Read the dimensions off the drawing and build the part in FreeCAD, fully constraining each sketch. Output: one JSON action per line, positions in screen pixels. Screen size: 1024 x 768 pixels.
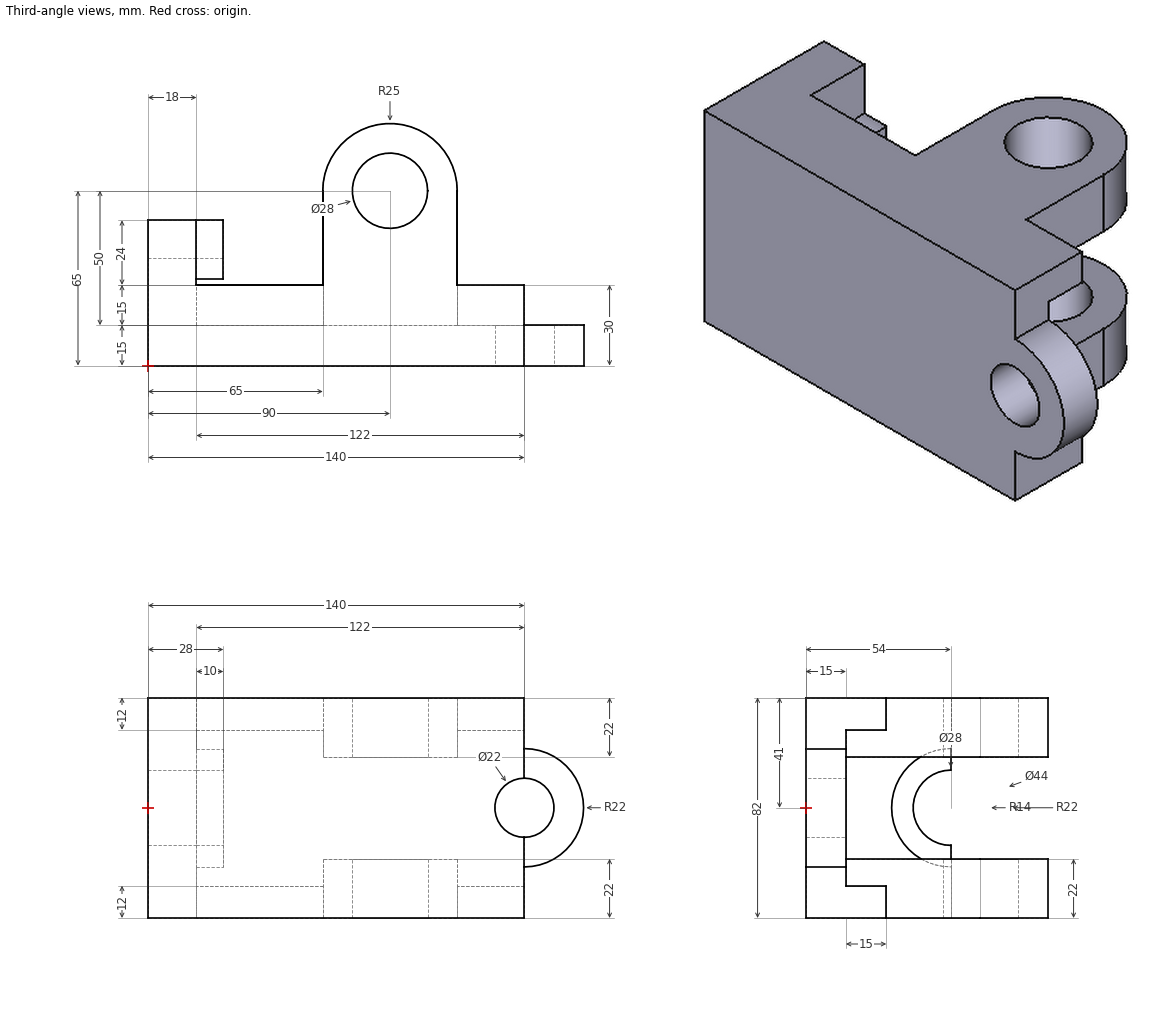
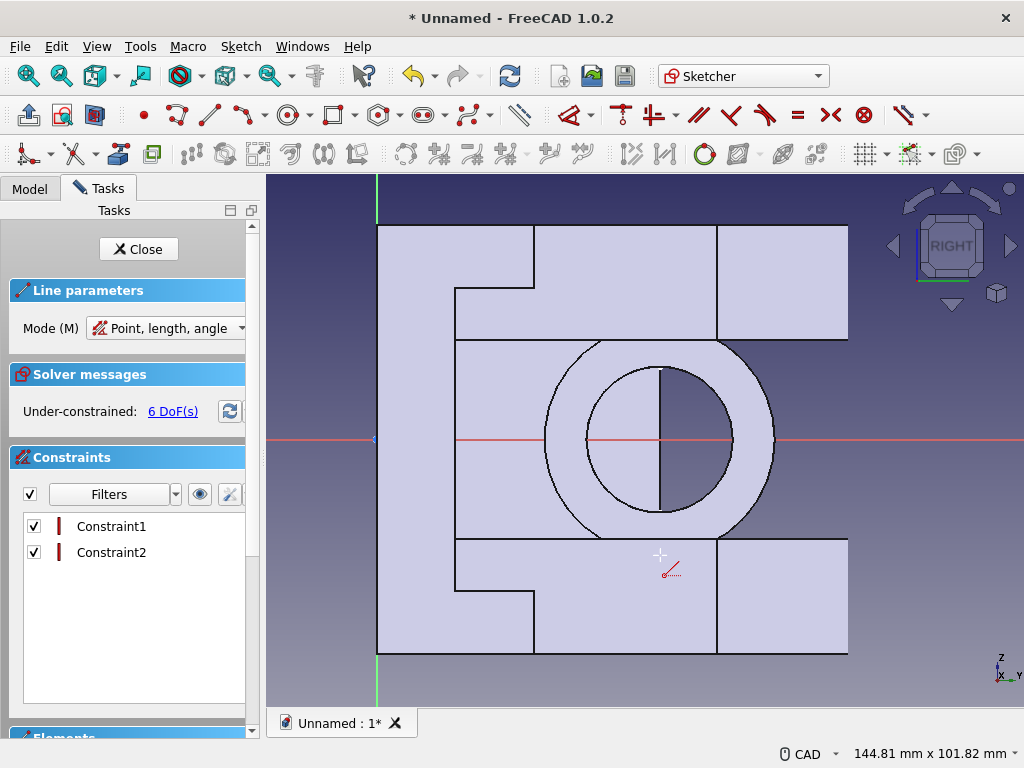
{"action": "key", "text": "g 3 a"}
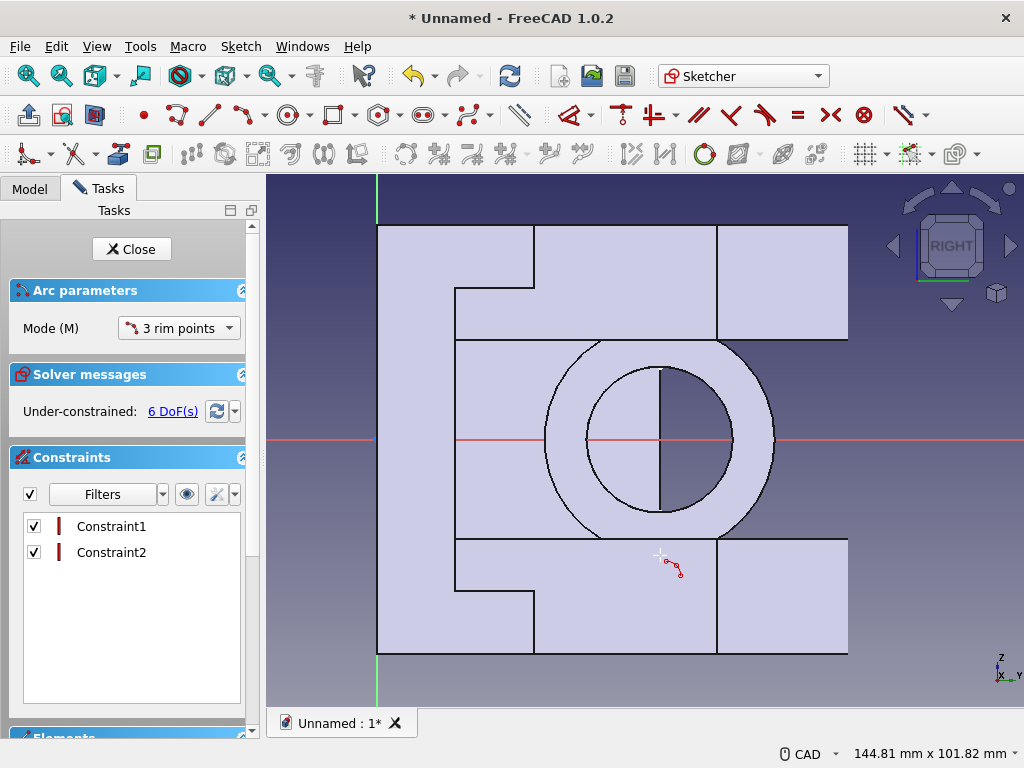
{"action": "left_click", "coordinate": [660, 367]}
{"action": "left_click", "coordinate": [660, 514]}
{"action": "left_click", "coordinate": [729, 462]}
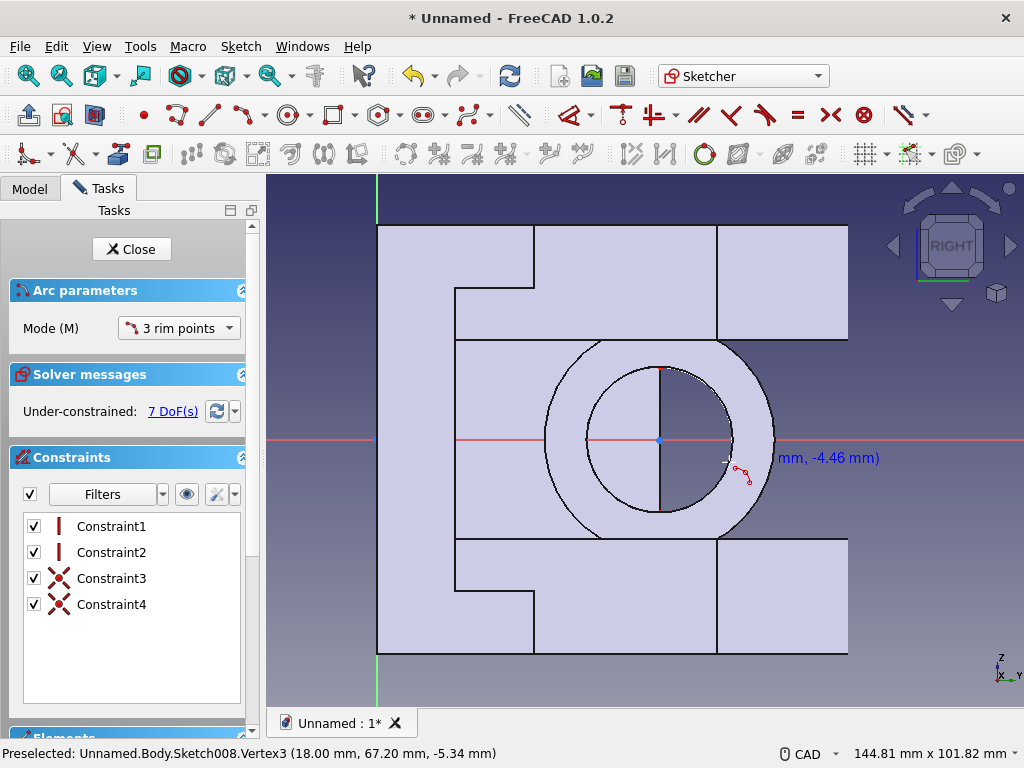
{"action": "left_click", "coordinate": [660, 556]}
{"action": "left_click", "coordinate": [660, 326]}
{"action": "left_click", "coordinate": [769, 475]}
{"action": "key", "text": "Escape"}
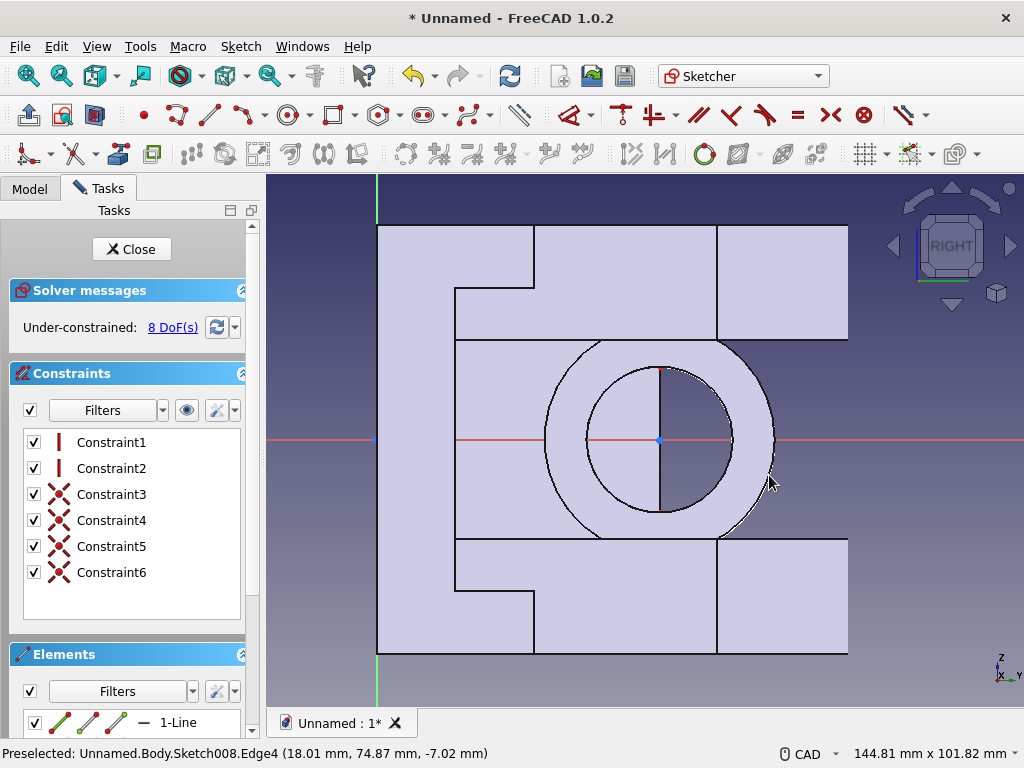
{"action": "left_click", "coordinate": [719, 483]}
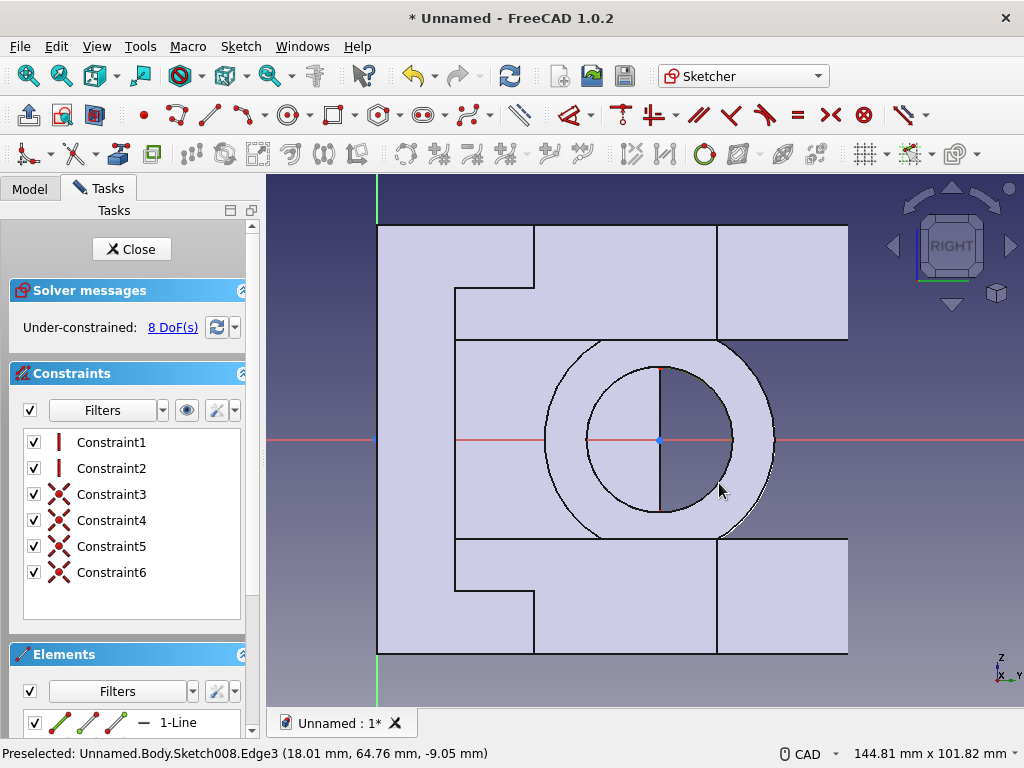
{"action": "left_click", "coordinate": [753, 508]}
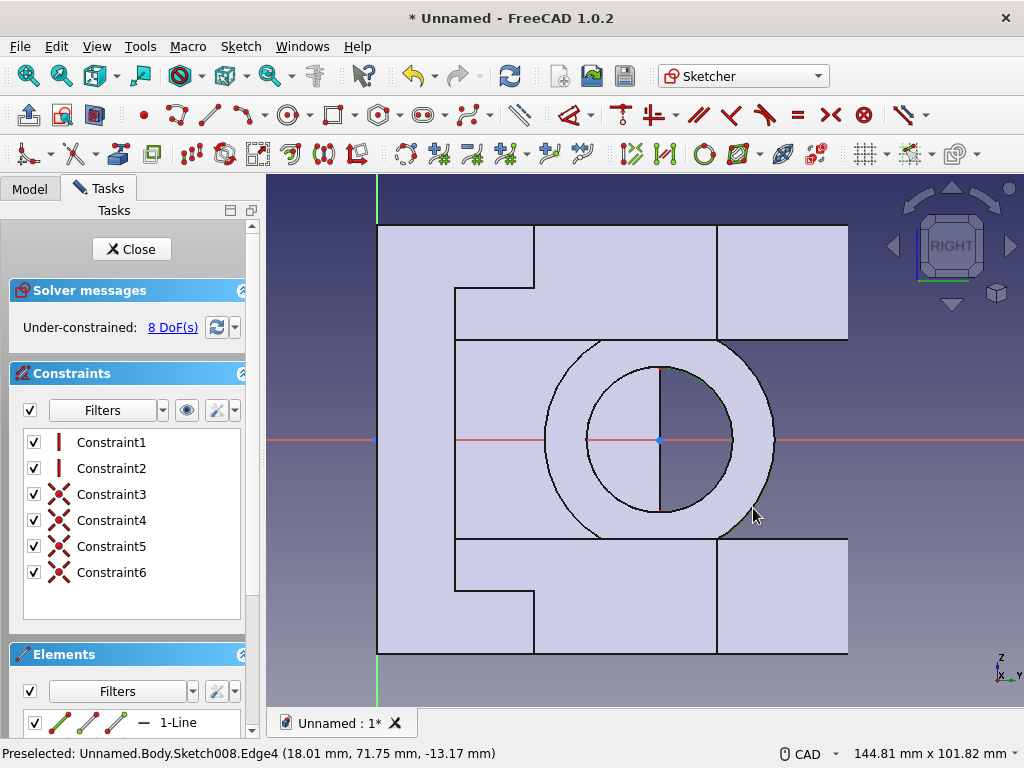
{"action": "key", "text": "c"}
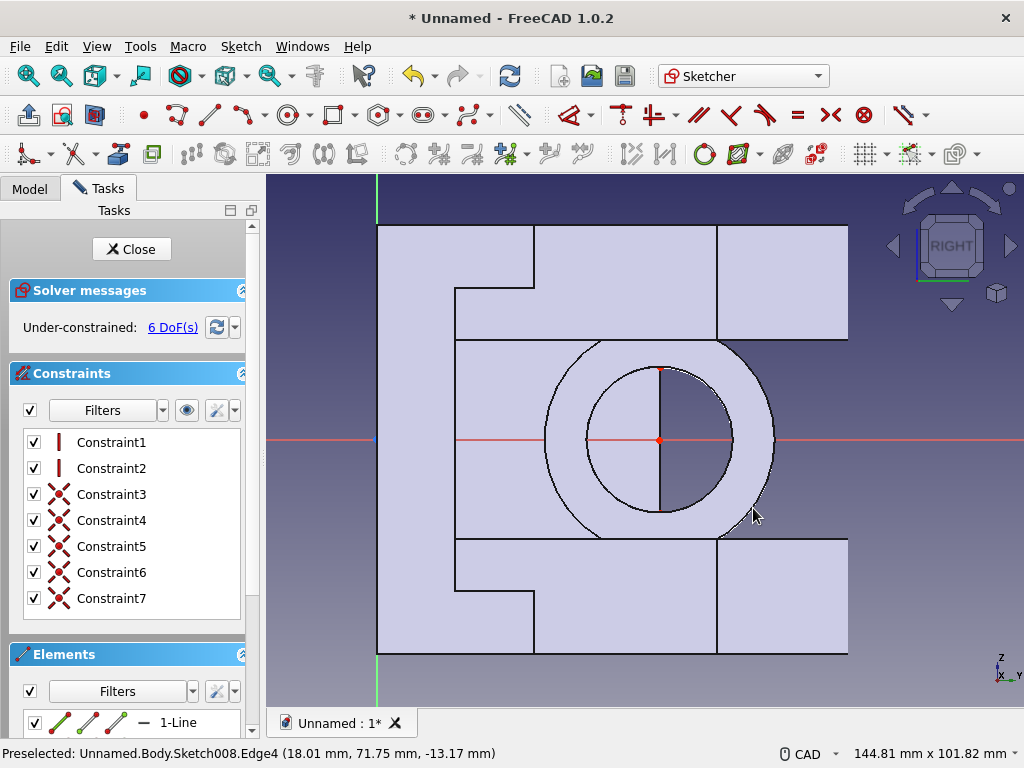
{"action": "left_click", "coordinate": [659, 441]}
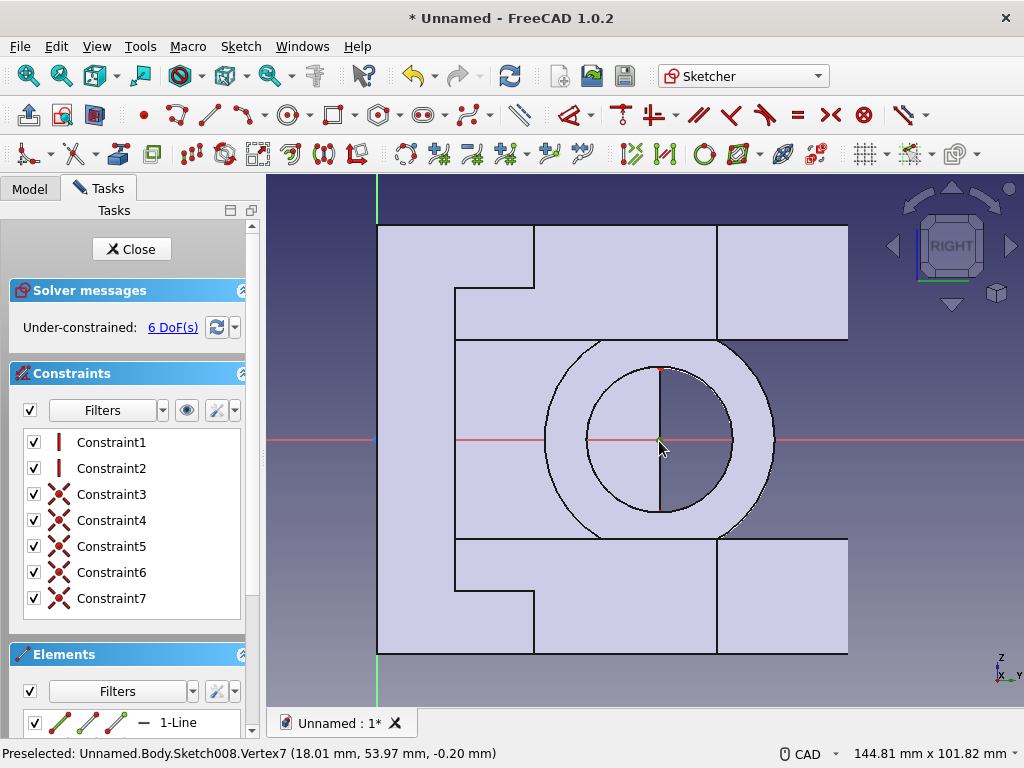
{"action": "left_click", "coordinate": [334, 440]}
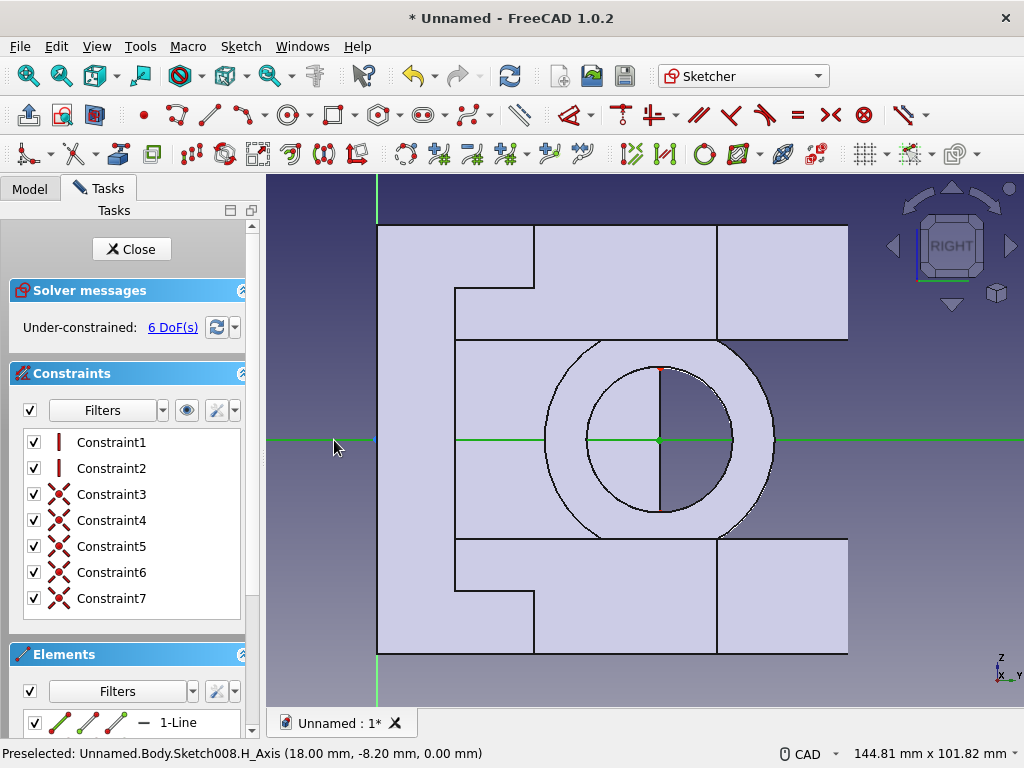
{"action": "left_click", "coordinate": [621, 116]}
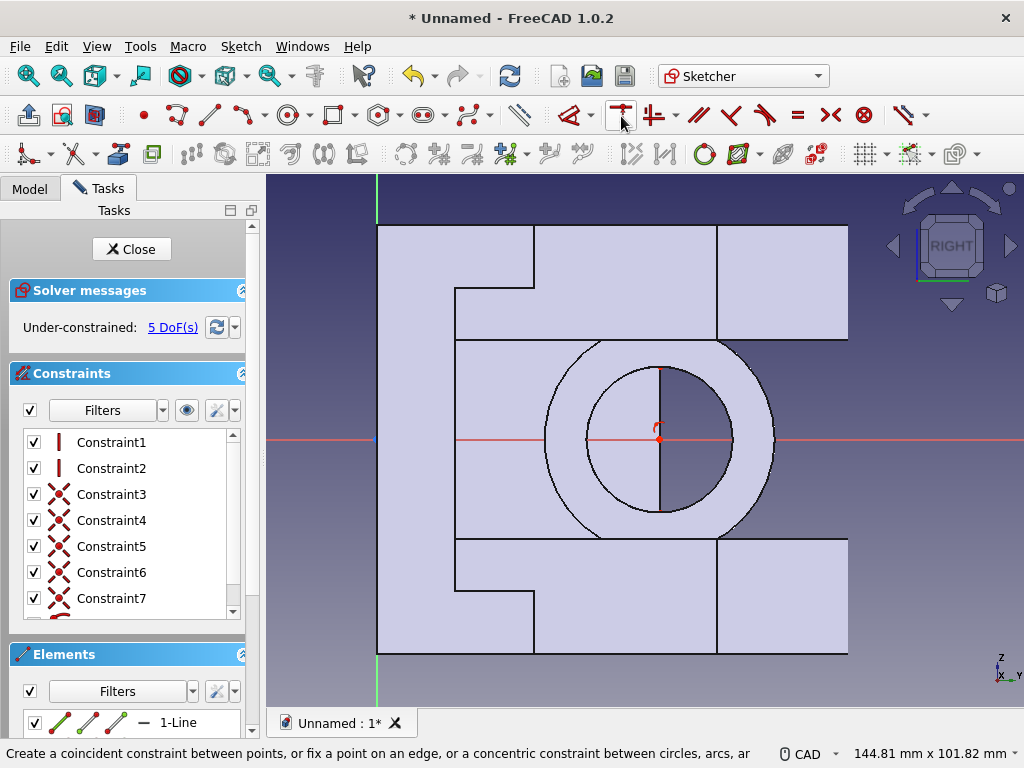
{"action": "key", "text": "d"}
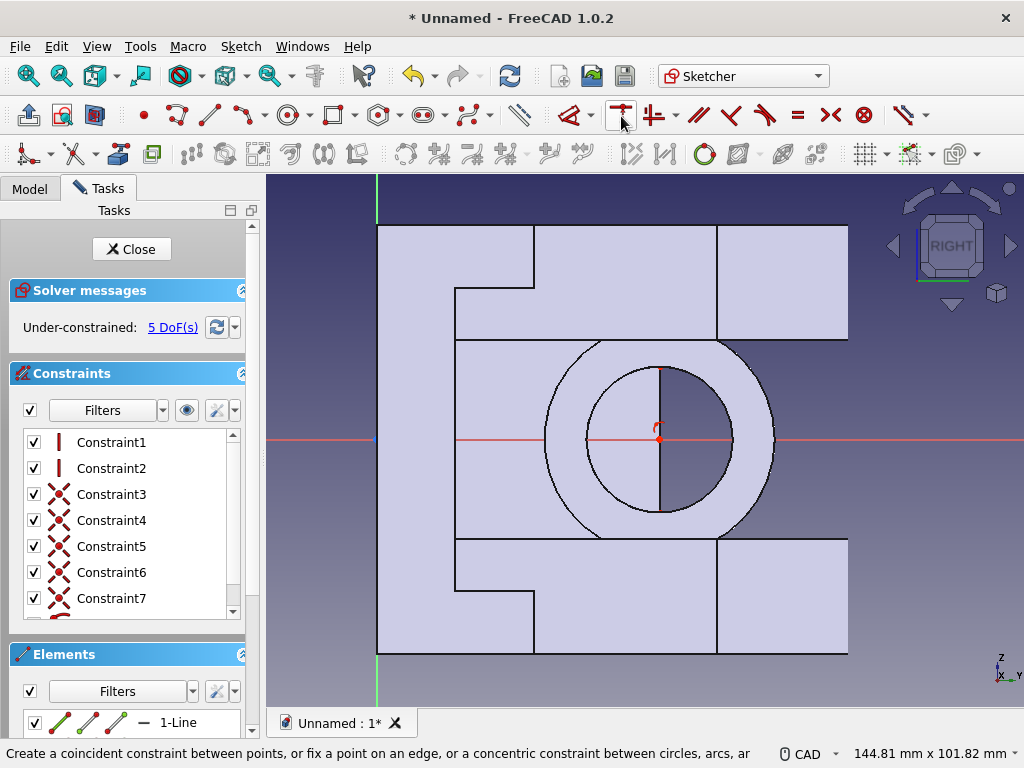
{"action": "left_click", "coordinate": [719, 483]}
{"action": "left_click", "coordinate": [597, 525]}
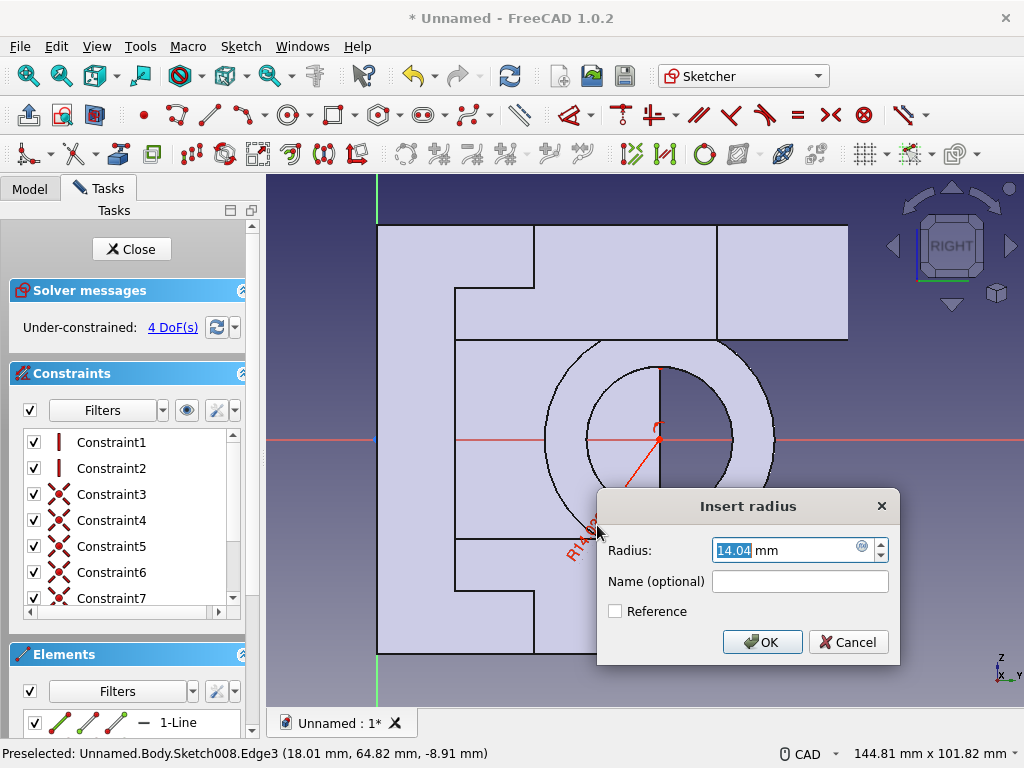
{"action": "type", "text": "14"}
{"action": "key", "text": "Return"}